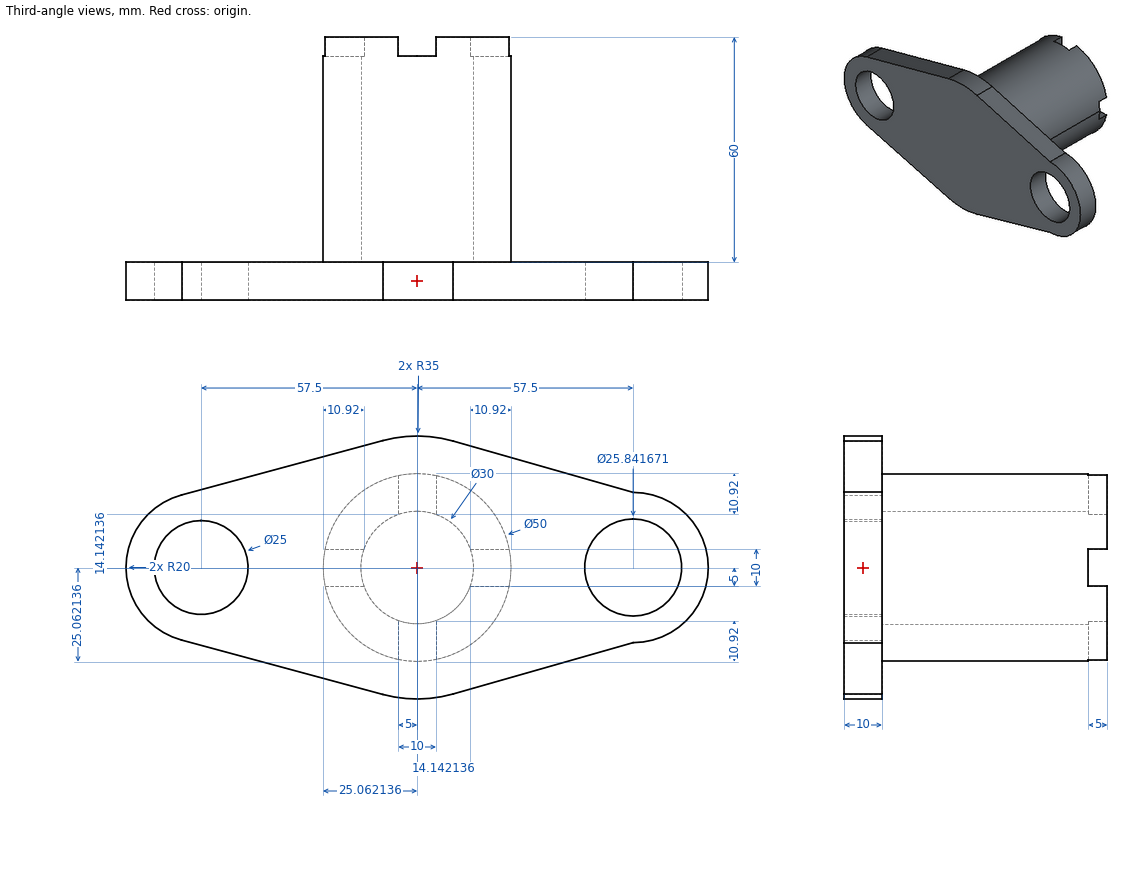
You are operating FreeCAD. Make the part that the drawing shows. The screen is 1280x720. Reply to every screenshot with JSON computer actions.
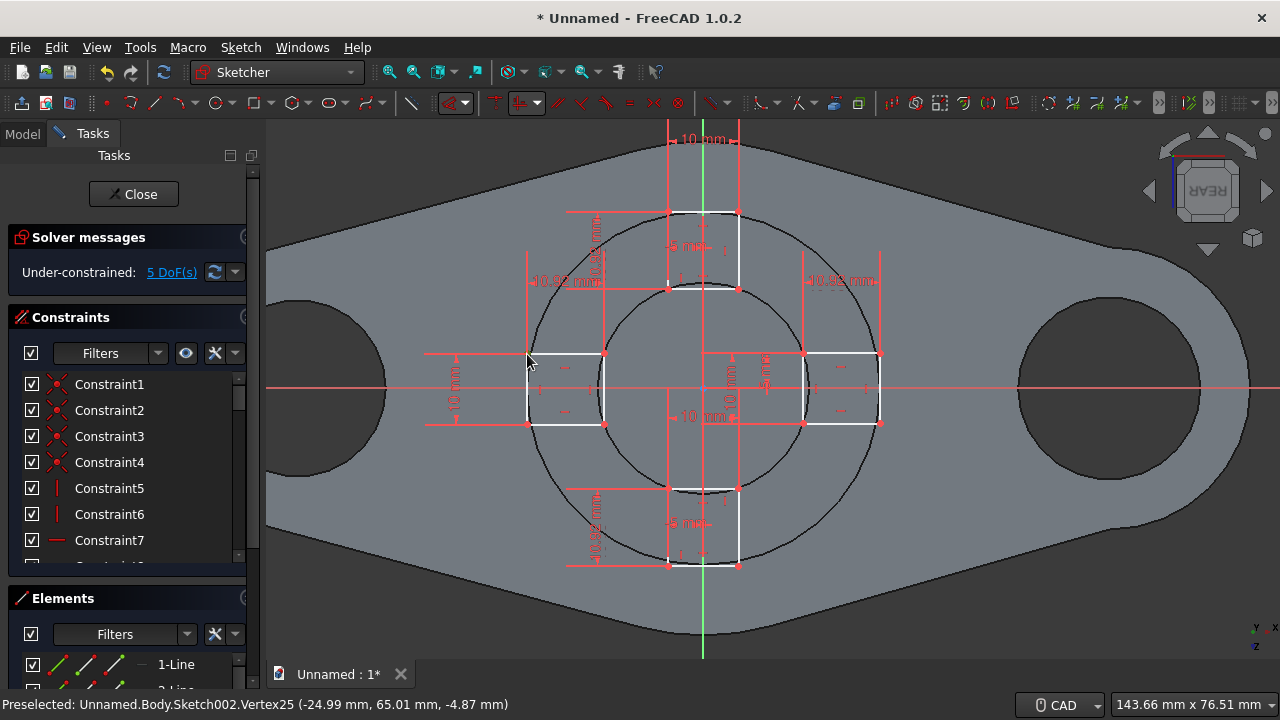
{"action": "key", "text": "i"}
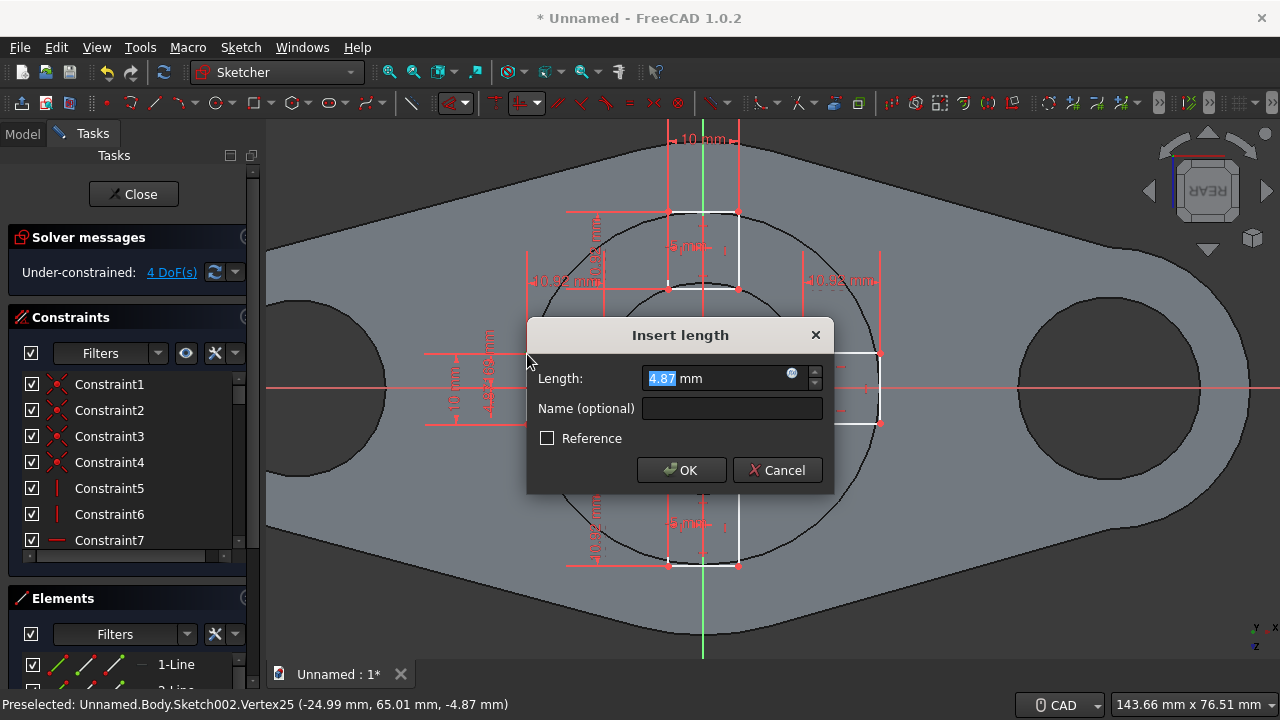
{"action": "type", "text": "5"}
{"action": "key", "text": "Return"}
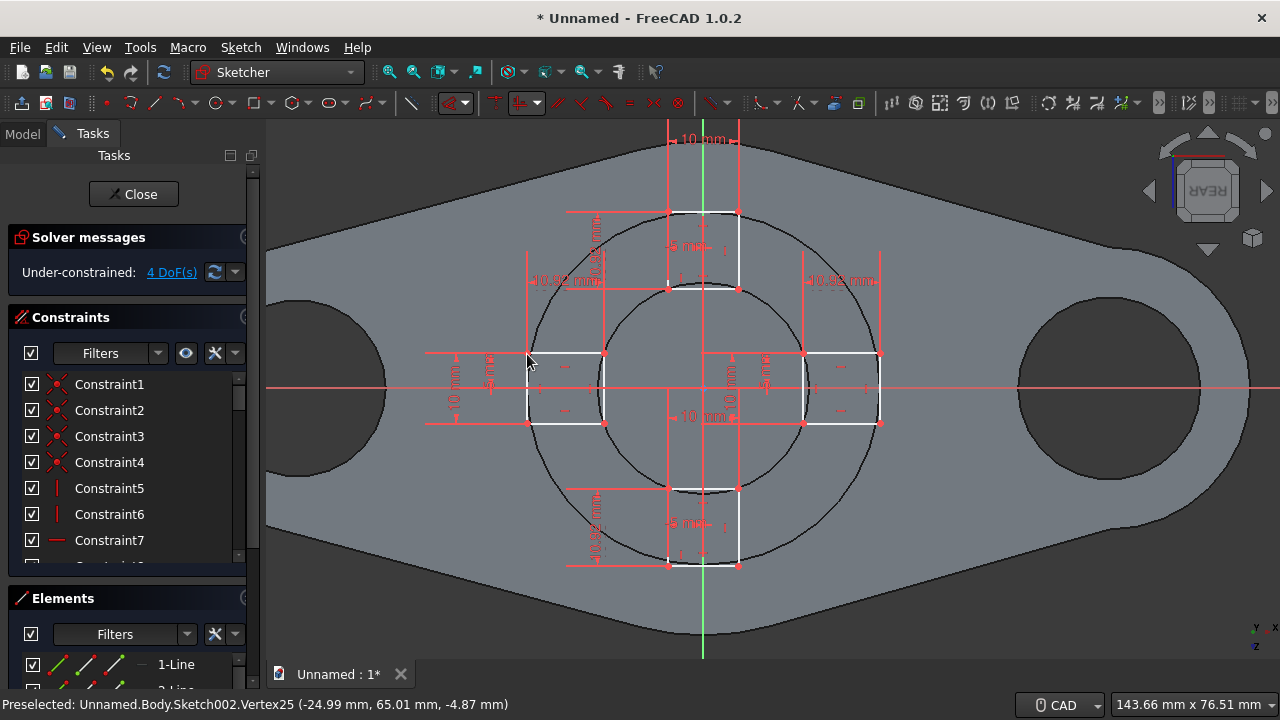
{"action": "left_click", "coordinate": [668, 212]}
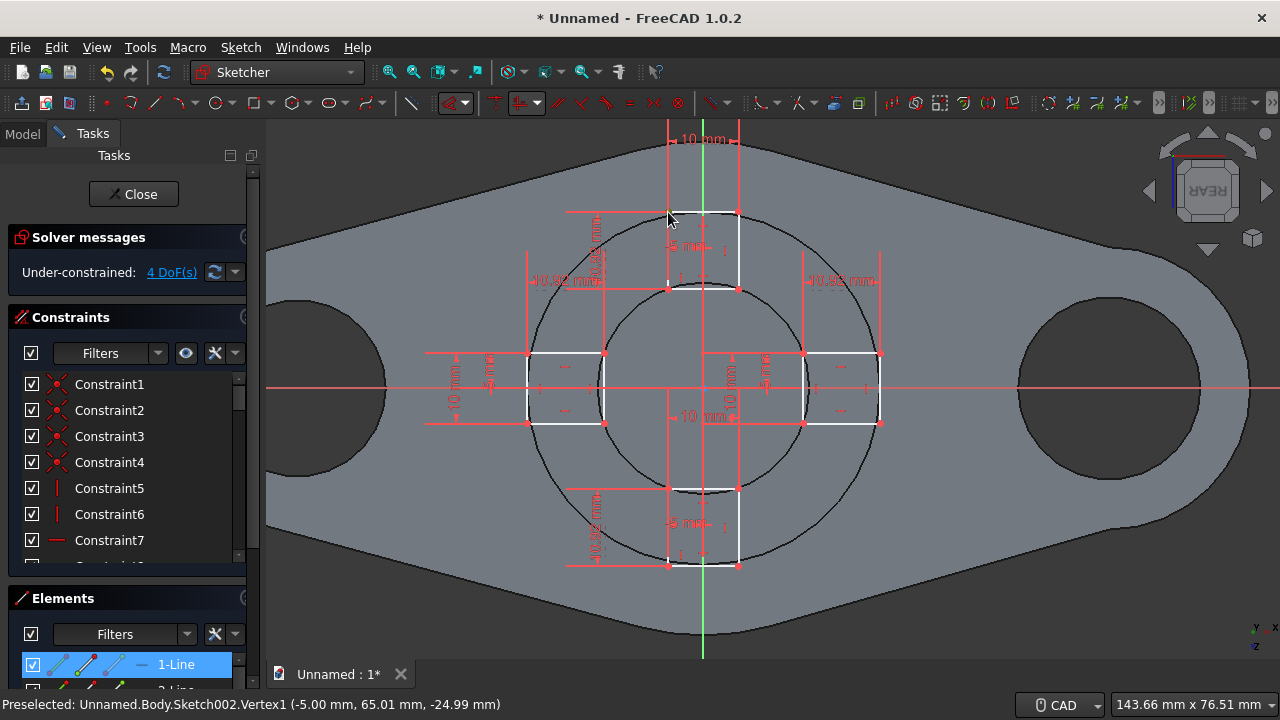
{"action": "key", "text": "i"}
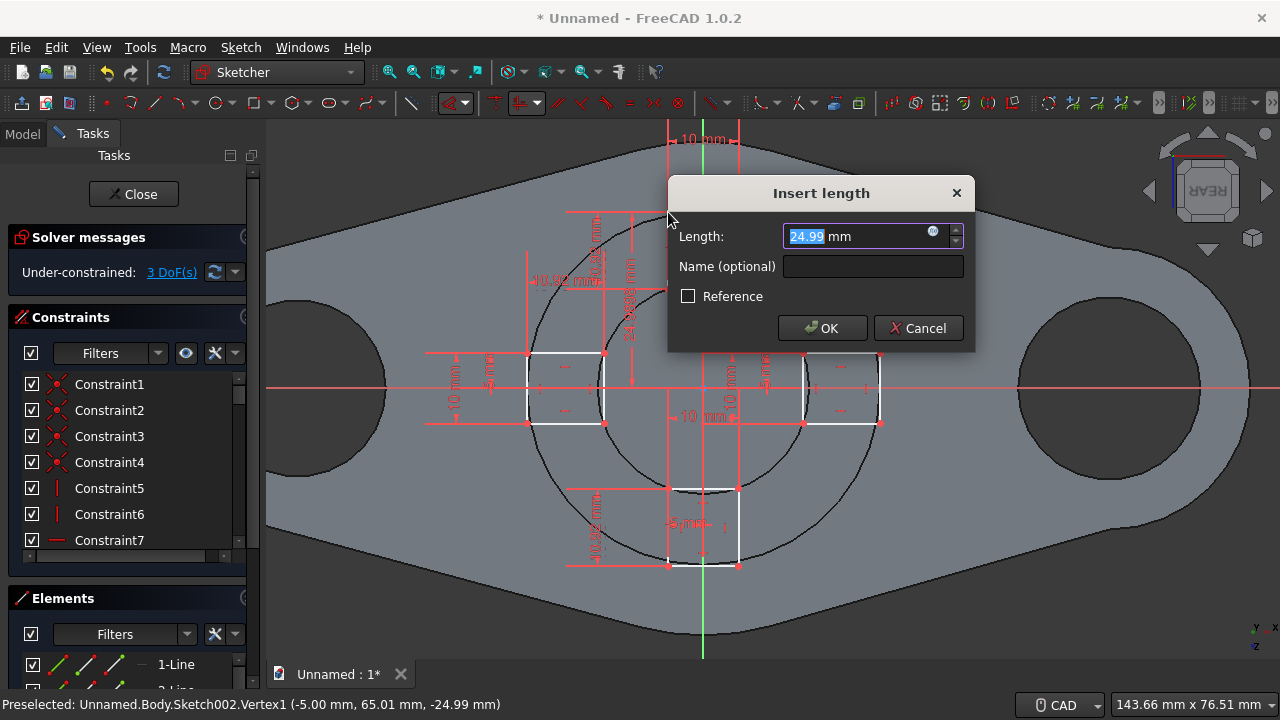
{"action": "type", "text": "25.062136"}
{"action": "key", "text": "Return"}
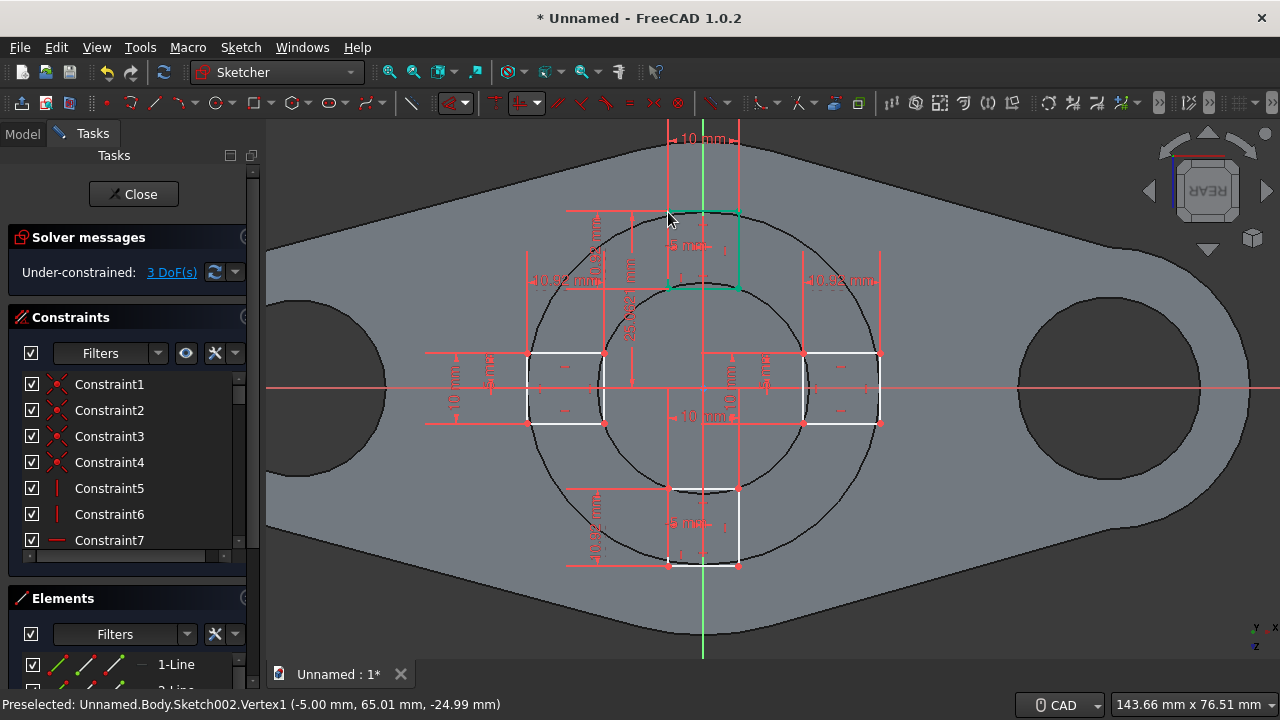
{"action": "left_click", "coordinate": [803, 353]}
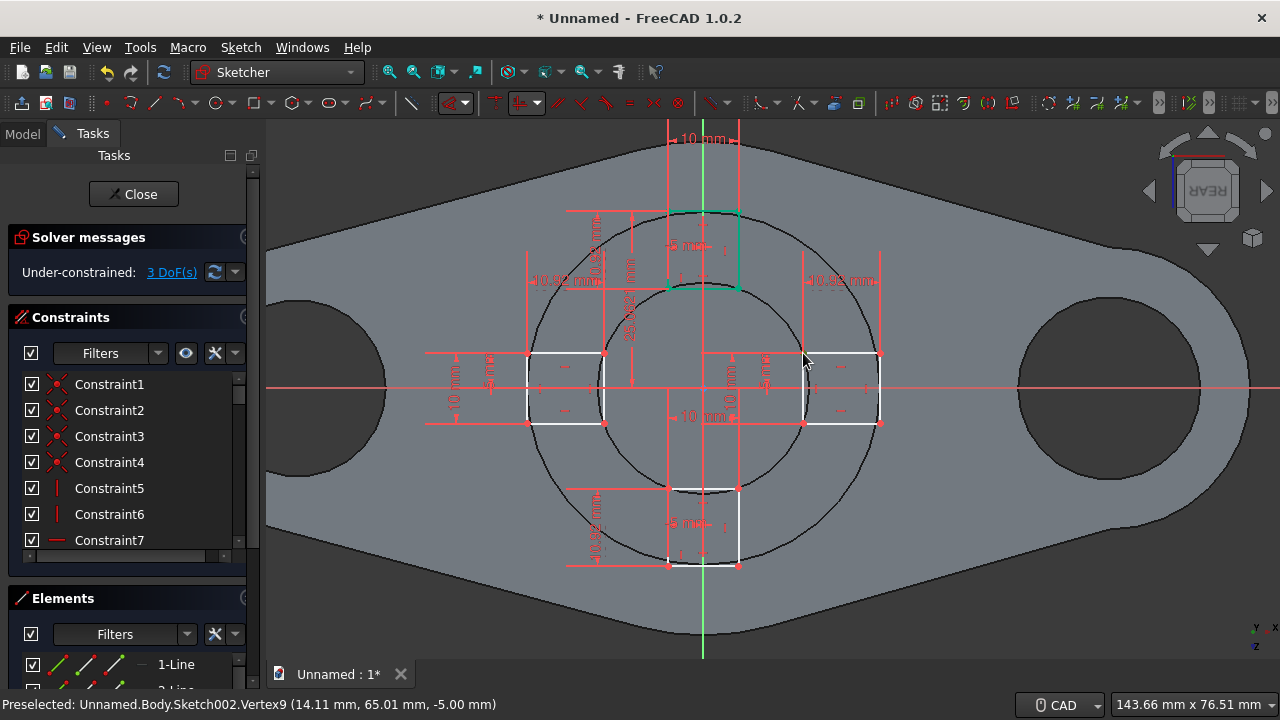
{"action": "key", "text": "l"}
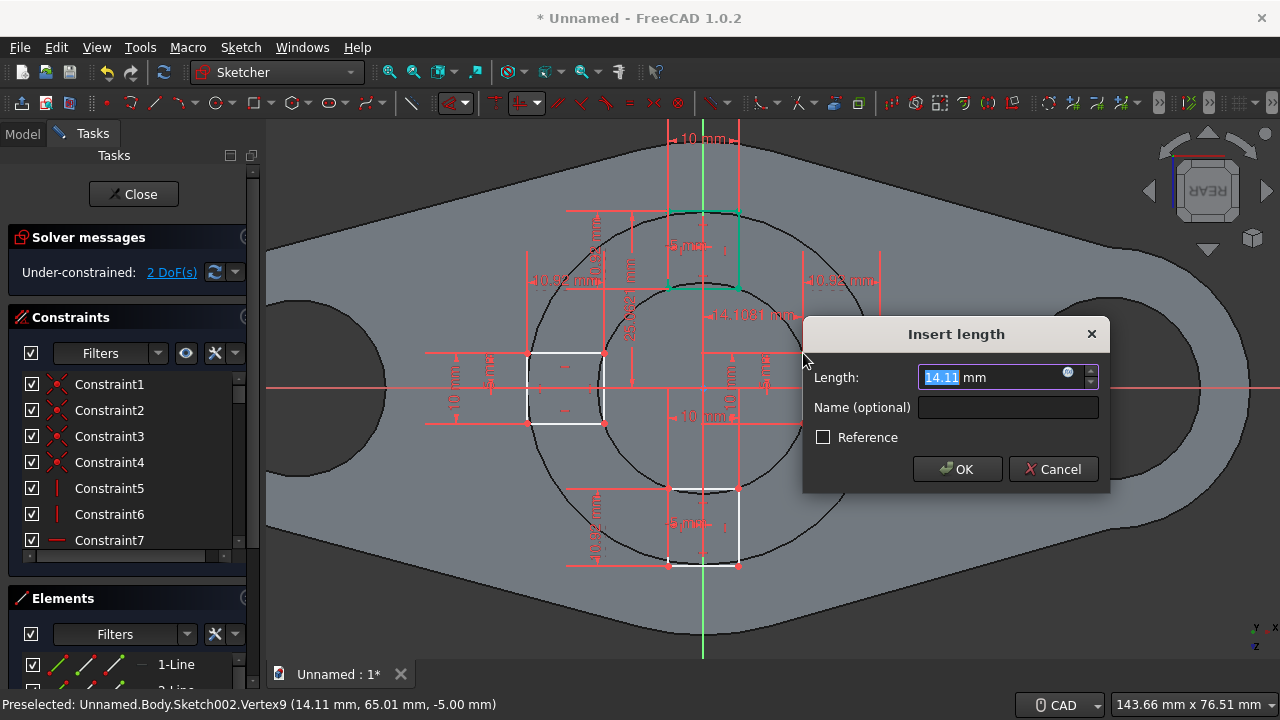
{"action": "type", "text": "14.142136"}
{"action": "key", "text": "Return"}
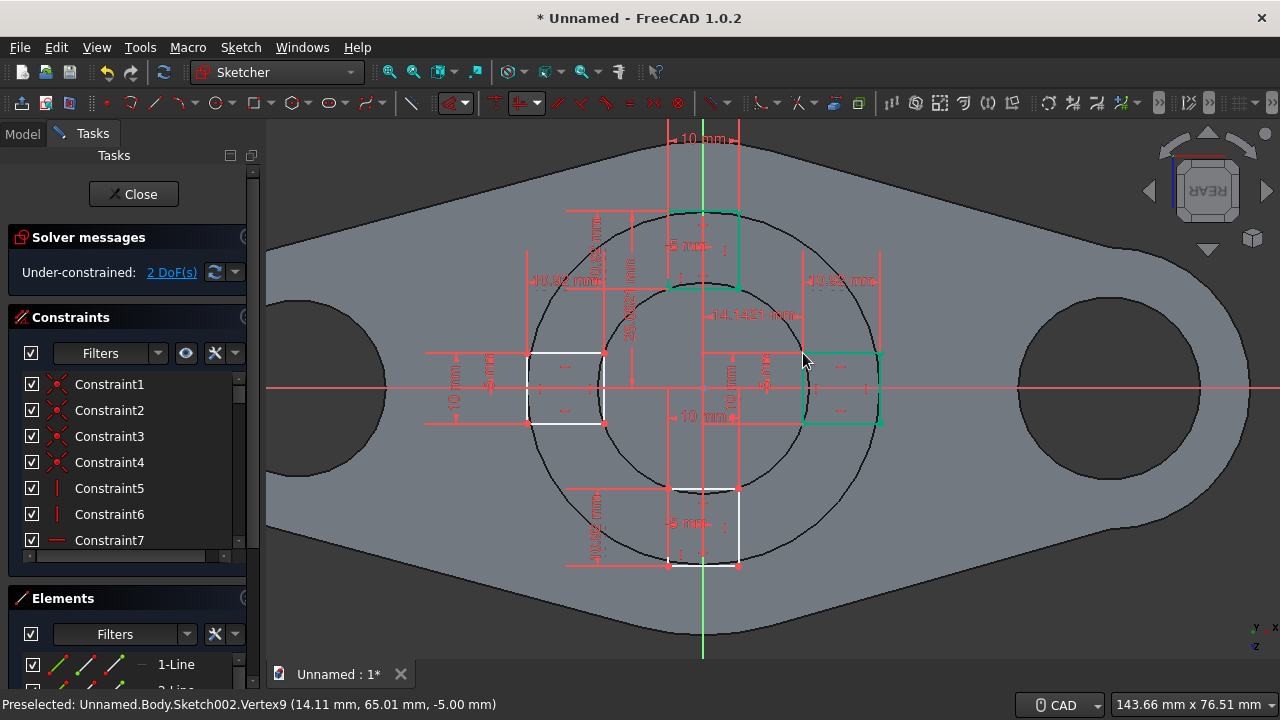
{"action": "left_click", "coordinate": [668, 489]}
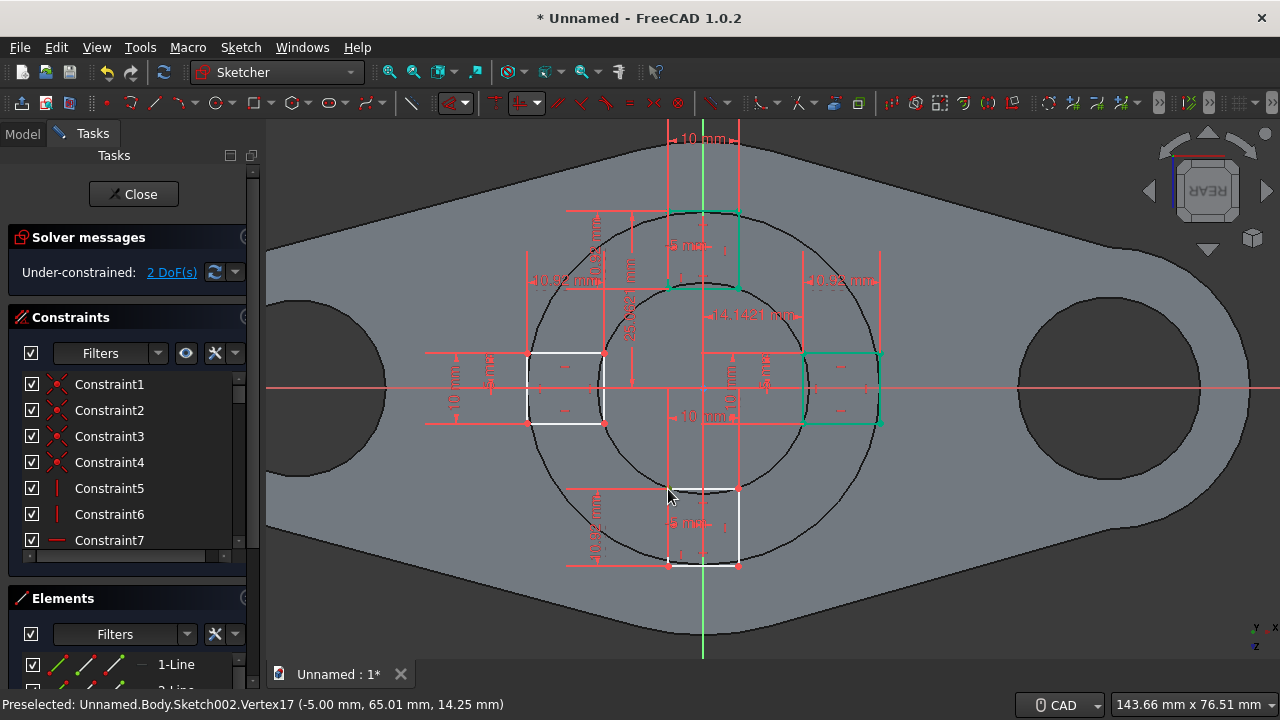
{"action": "key", "text": "i"}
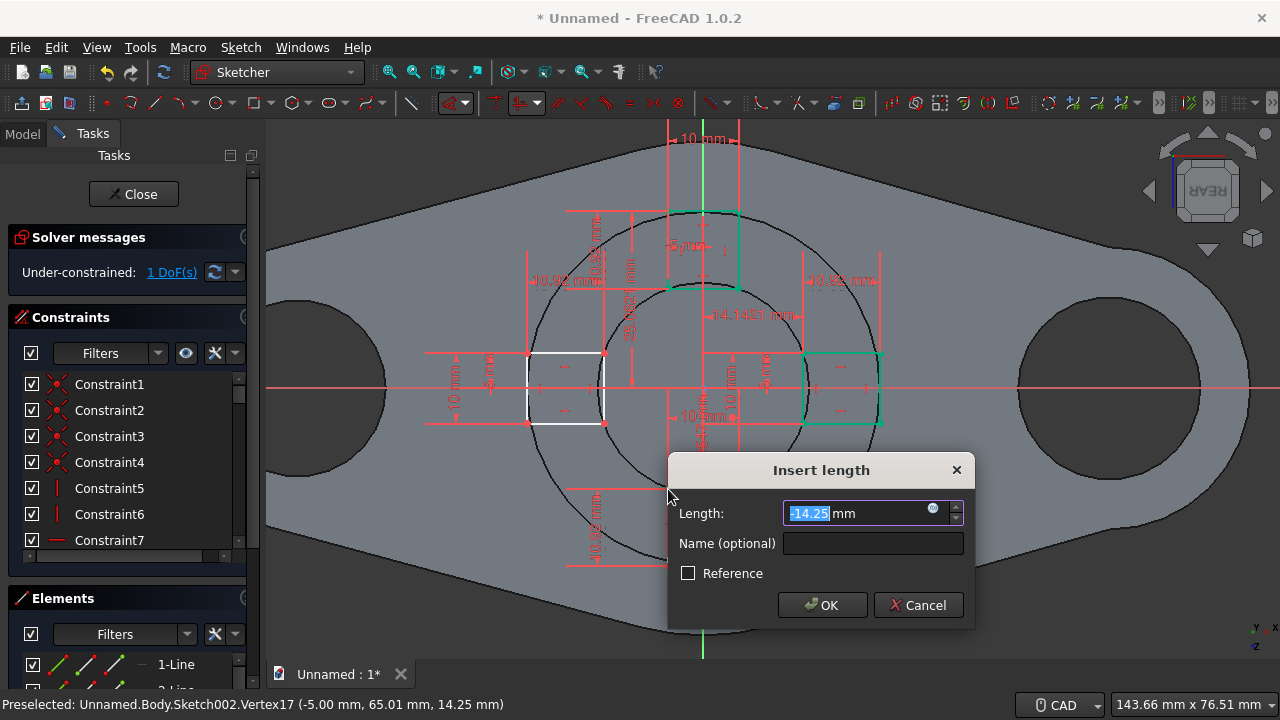
{"action": "type", "text": "-14.142136"}
{"action": "key", "text": "Return"}